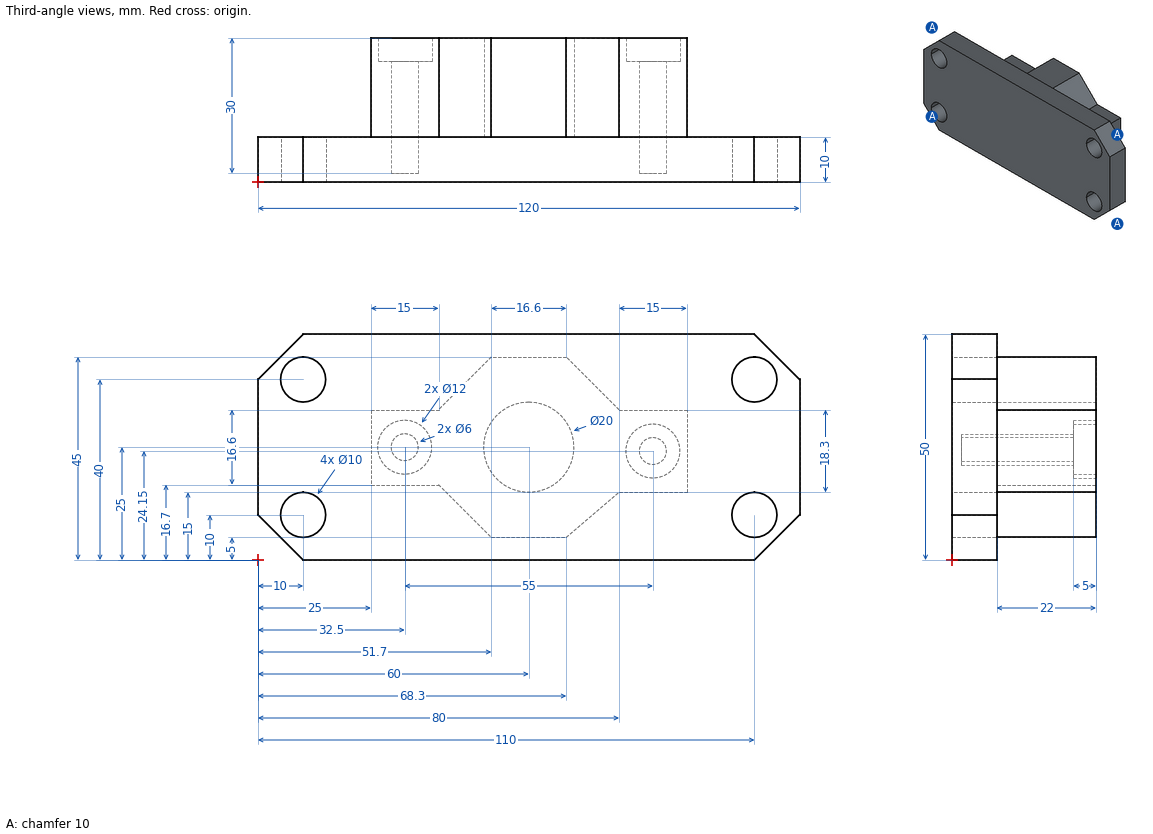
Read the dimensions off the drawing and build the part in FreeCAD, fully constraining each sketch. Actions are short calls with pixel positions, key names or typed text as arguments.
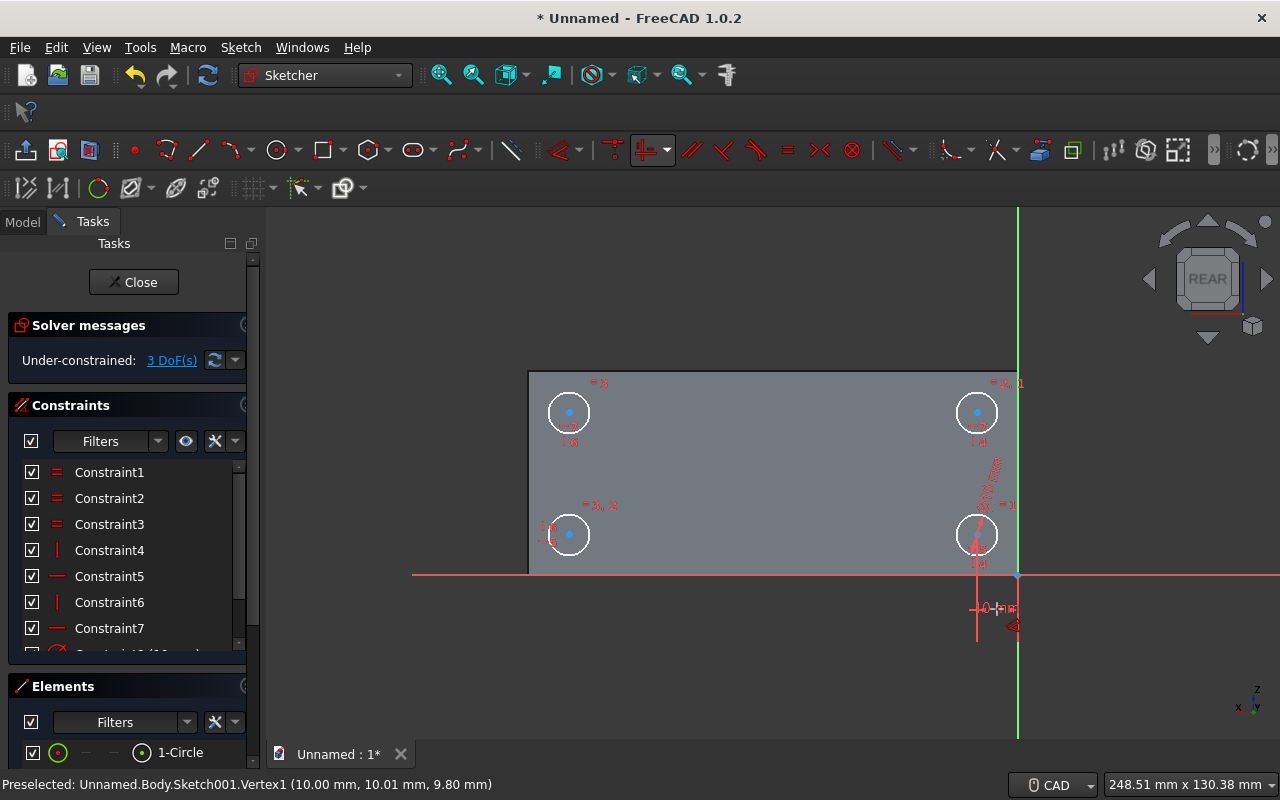
click(977, 535)
click(1052, 555)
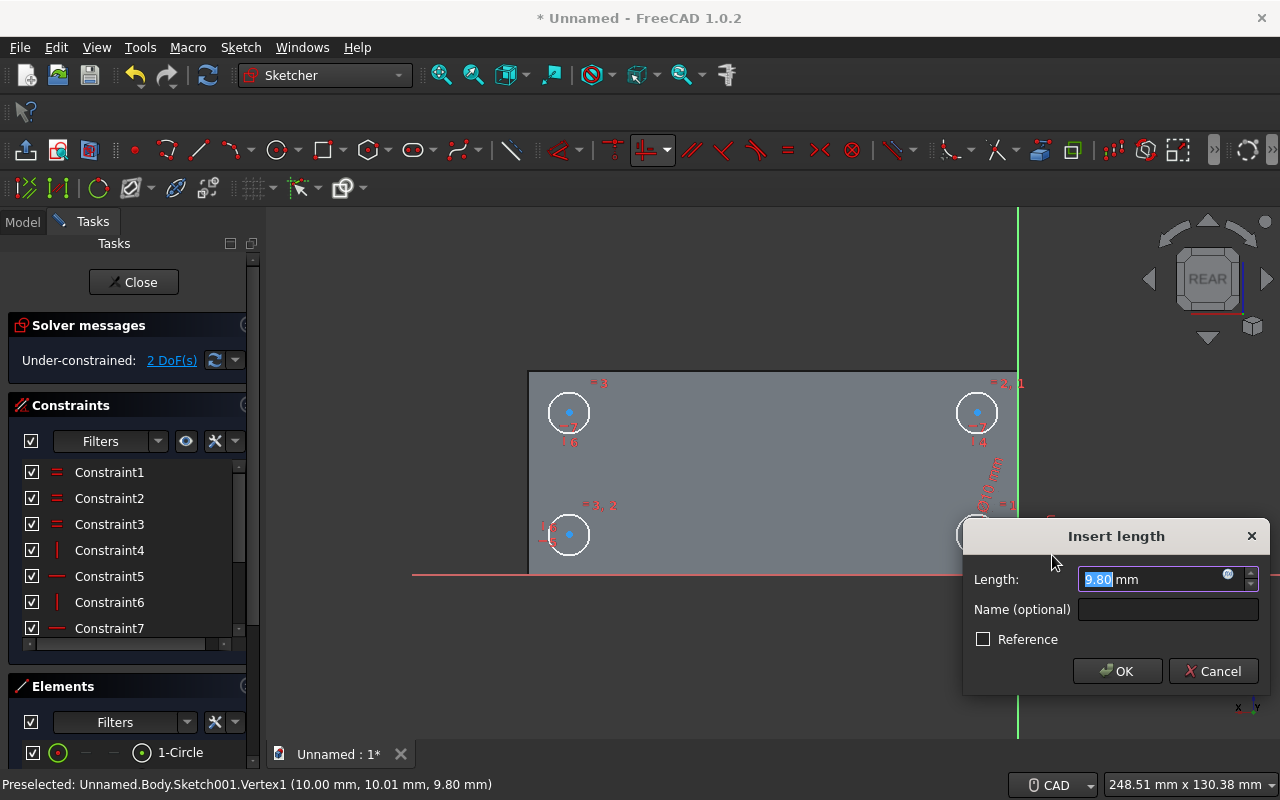
text(10)
key(Return)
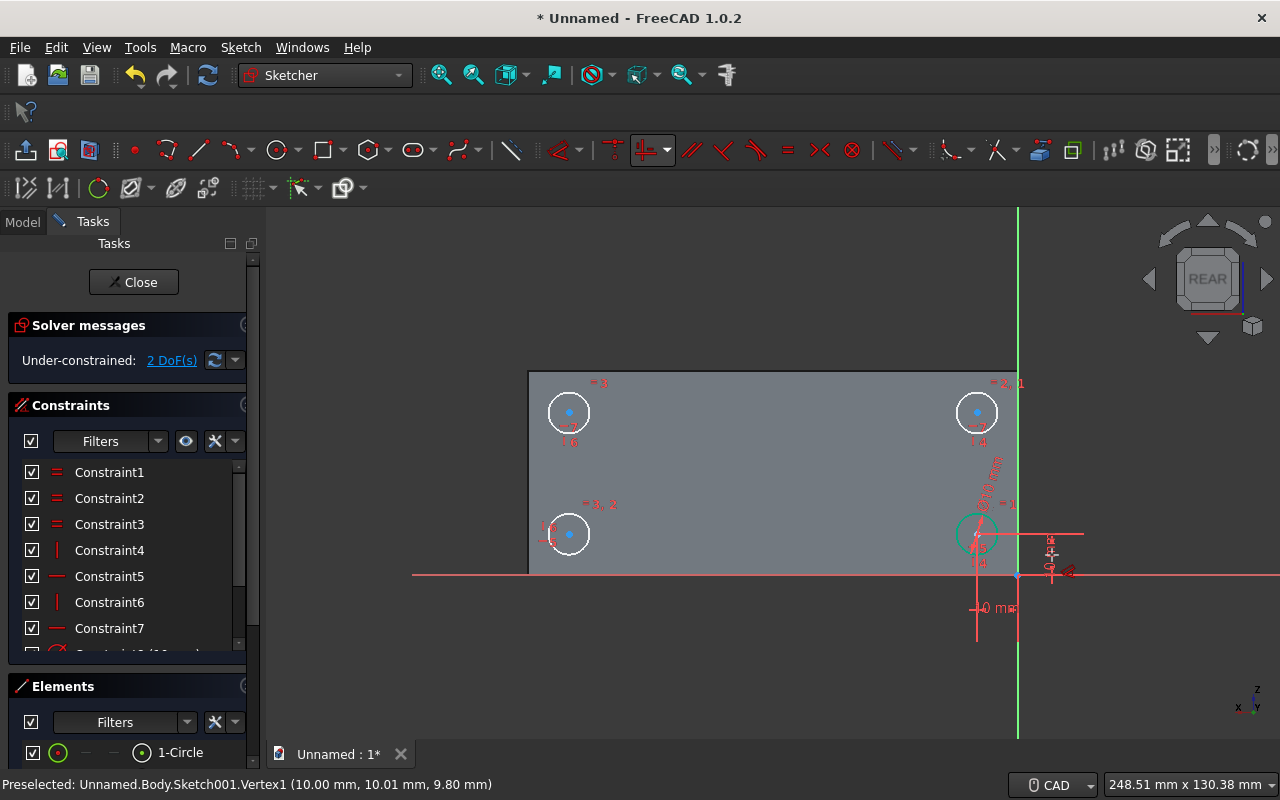
click(977, 413)
click(1052, 457)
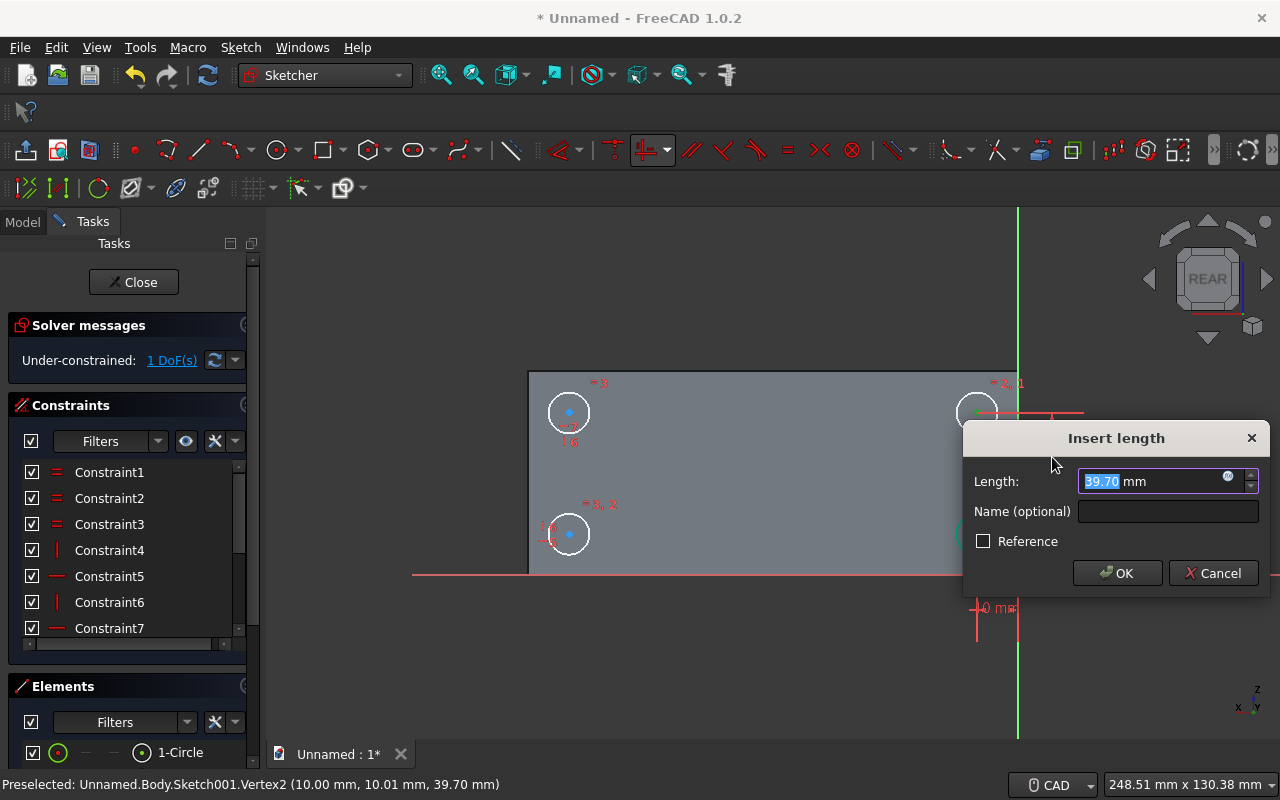
text(40)
key(Return)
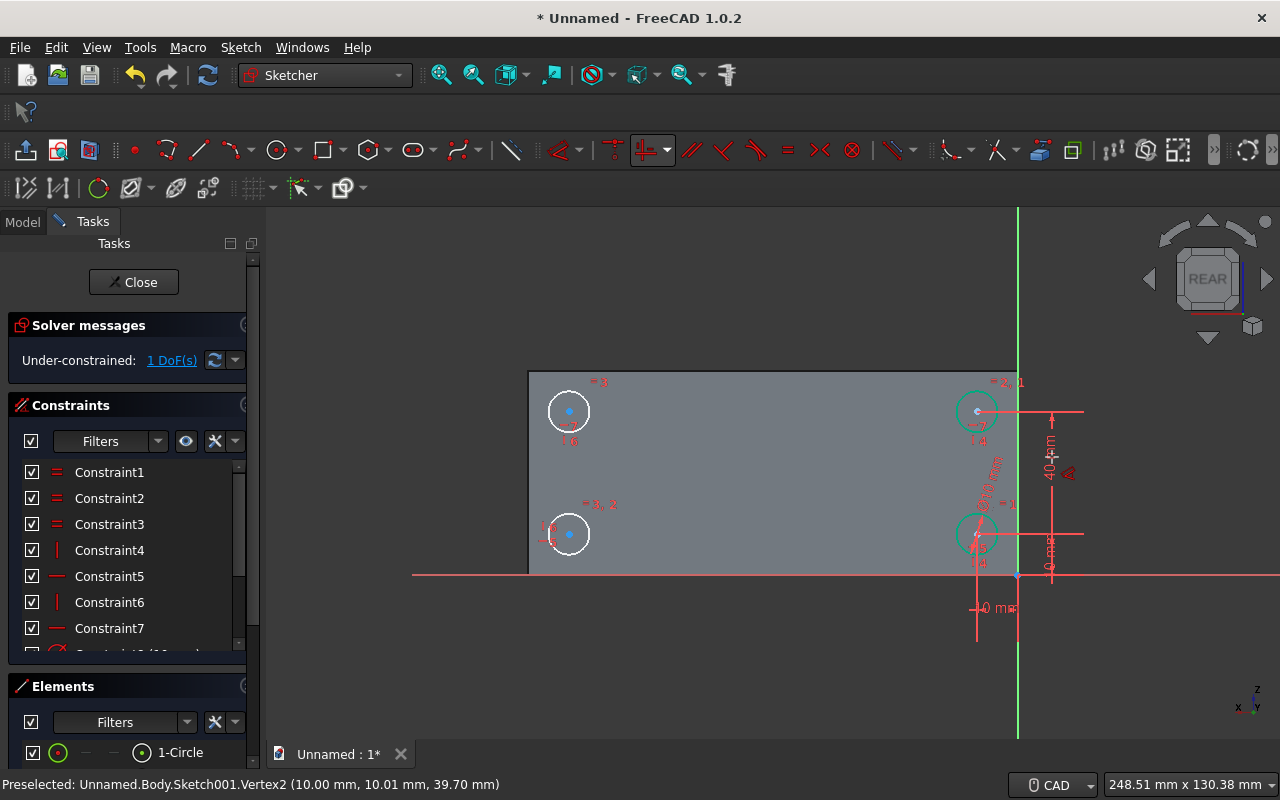
click(569, 534)
click(793, 609)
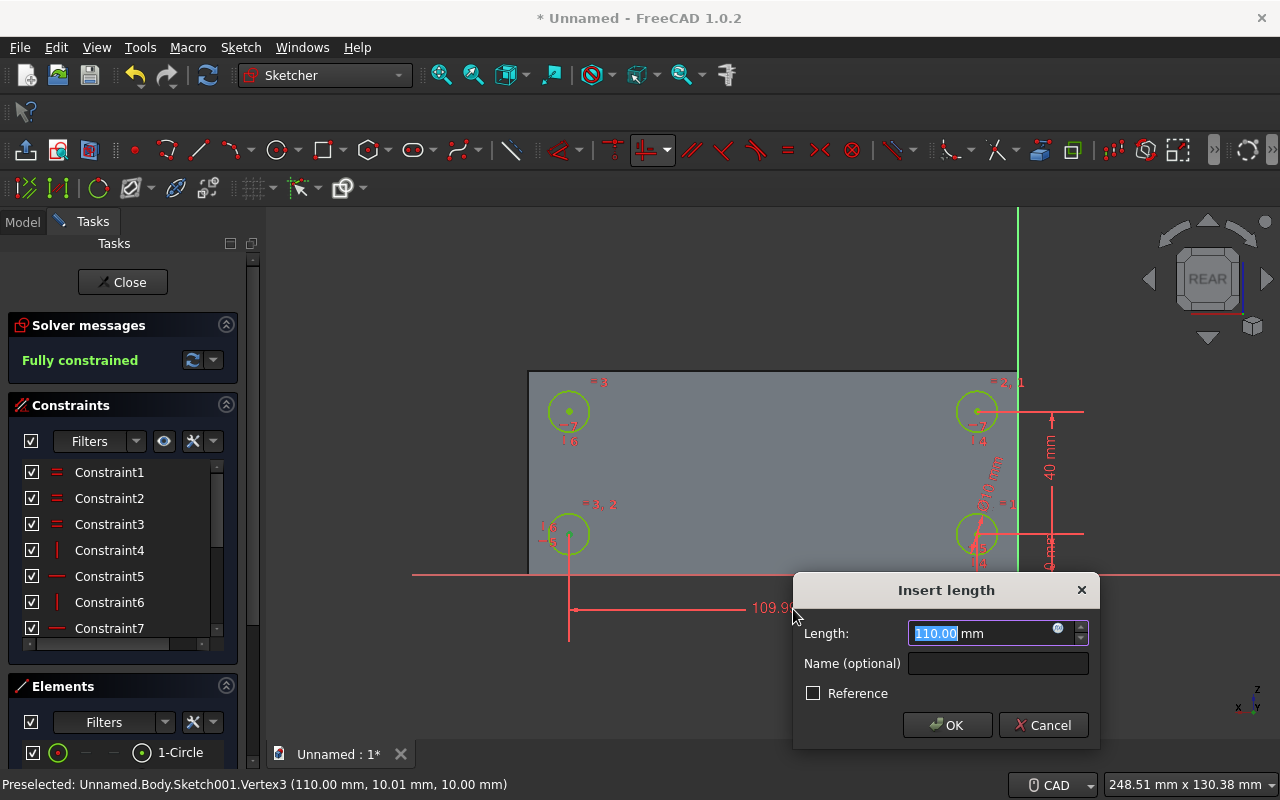
text(110)
key(Return)
key(Escape)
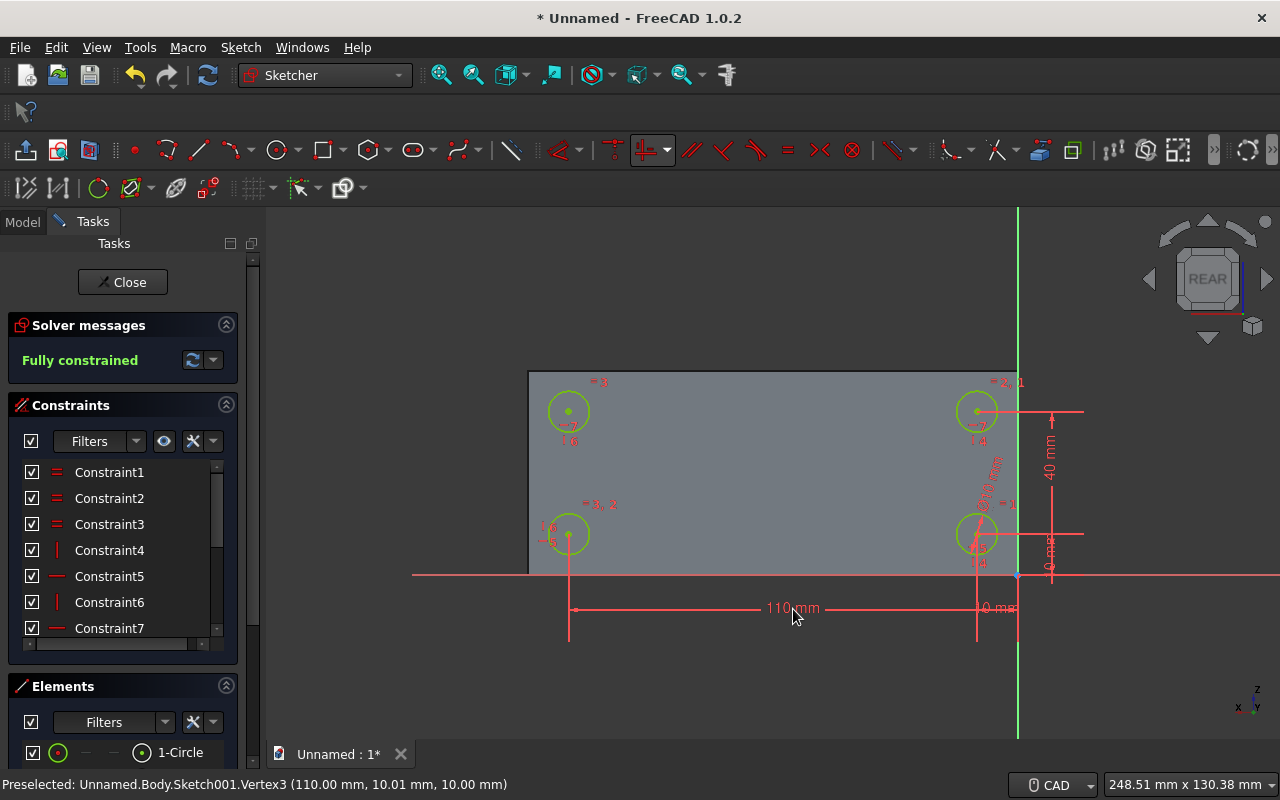
click(123, 282)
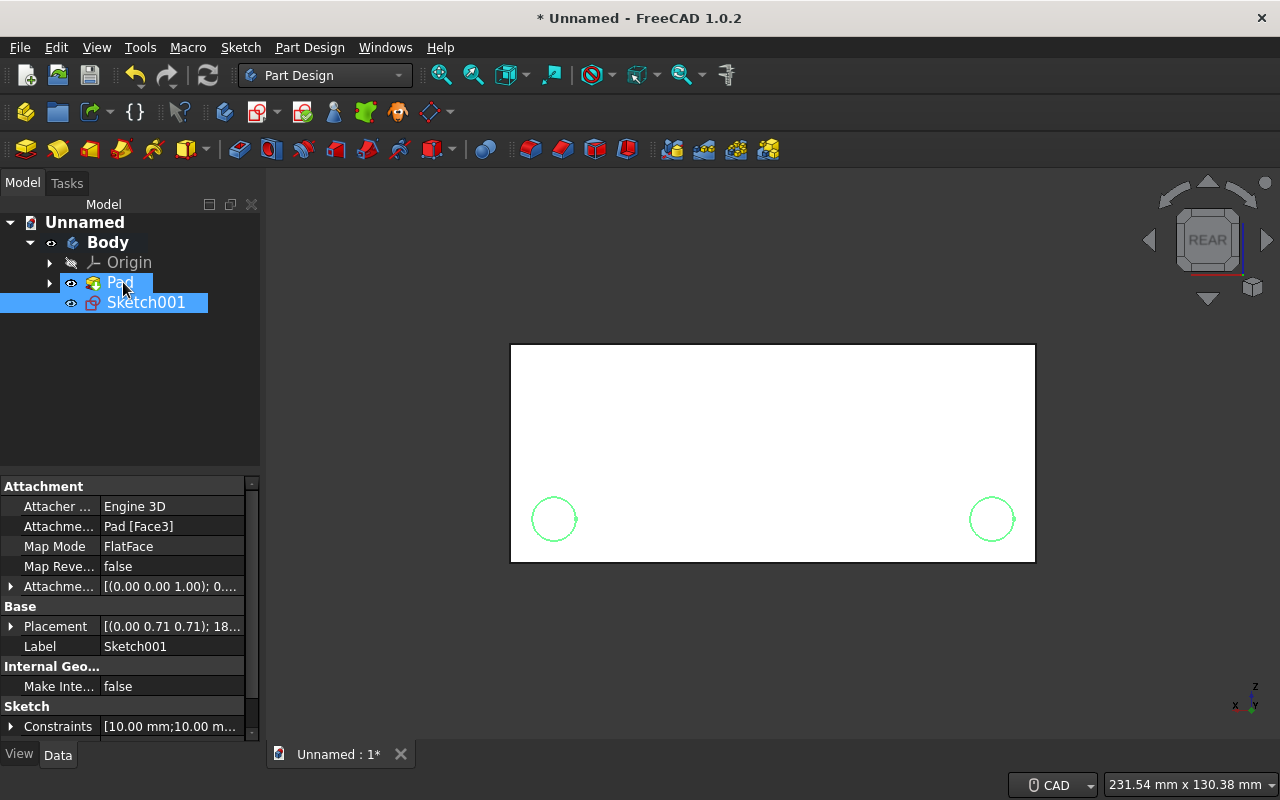
click(240, 150)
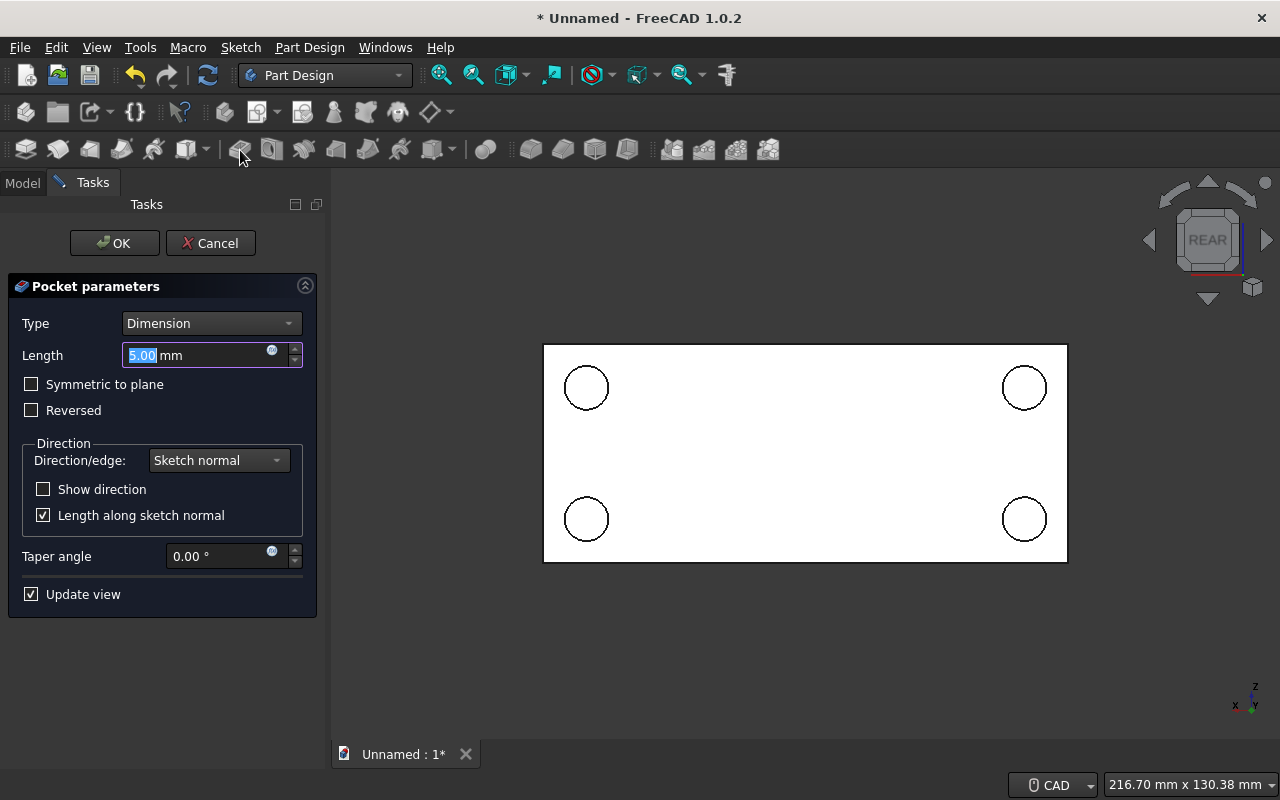
click(212, 324)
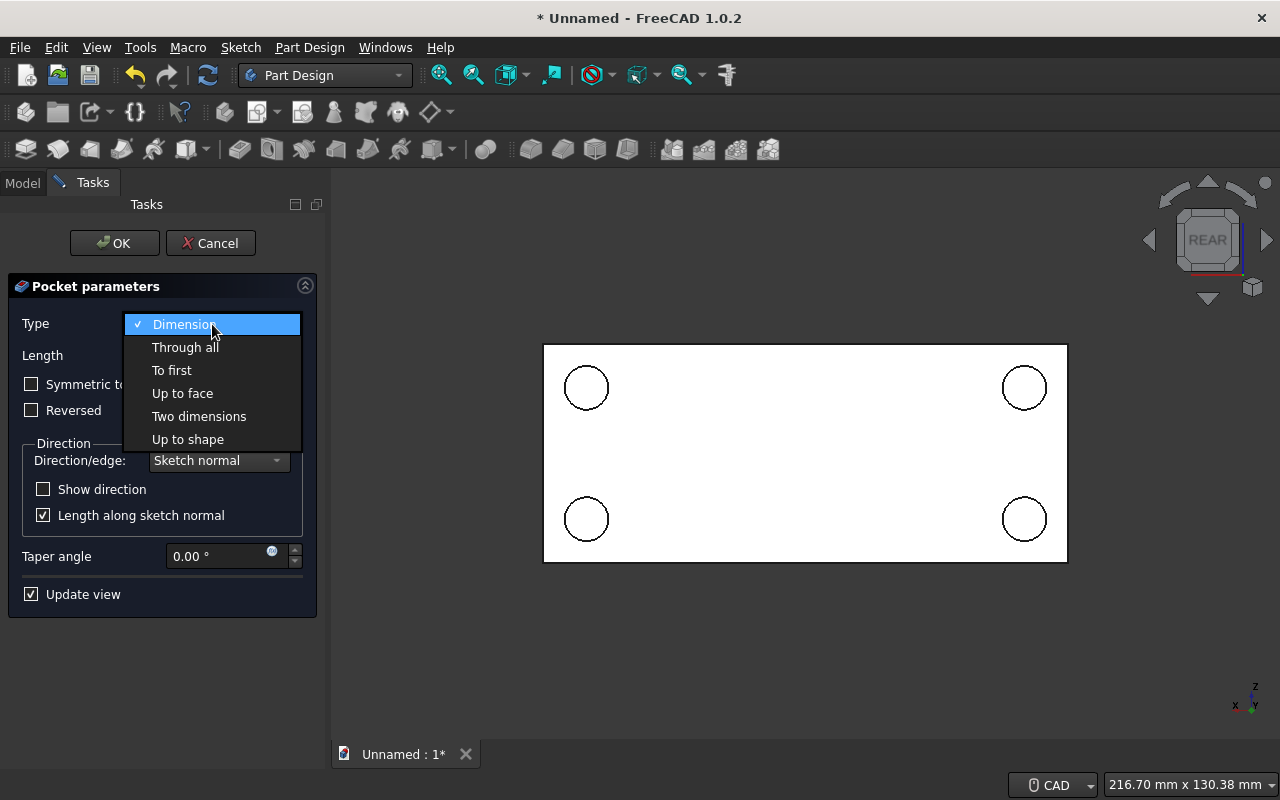
click(212, 348)